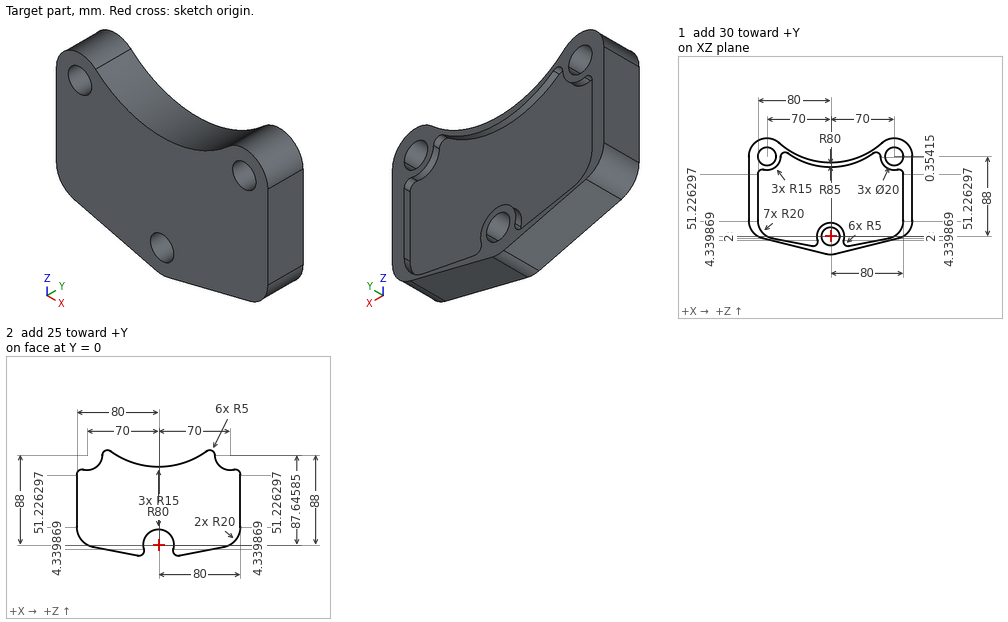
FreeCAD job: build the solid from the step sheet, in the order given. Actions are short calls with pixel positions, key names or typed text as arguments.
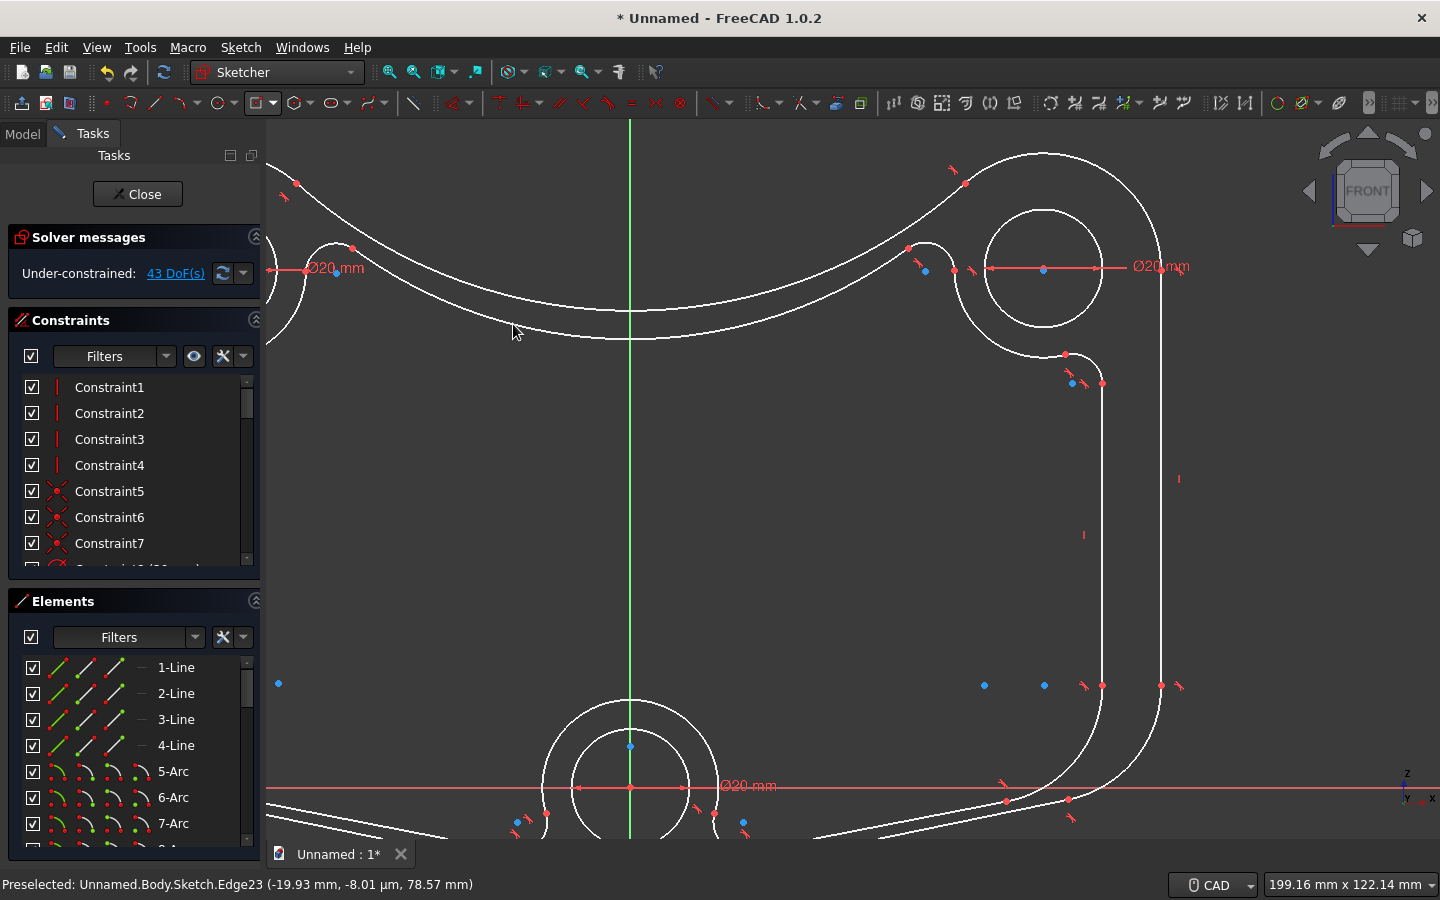
click(513, 324)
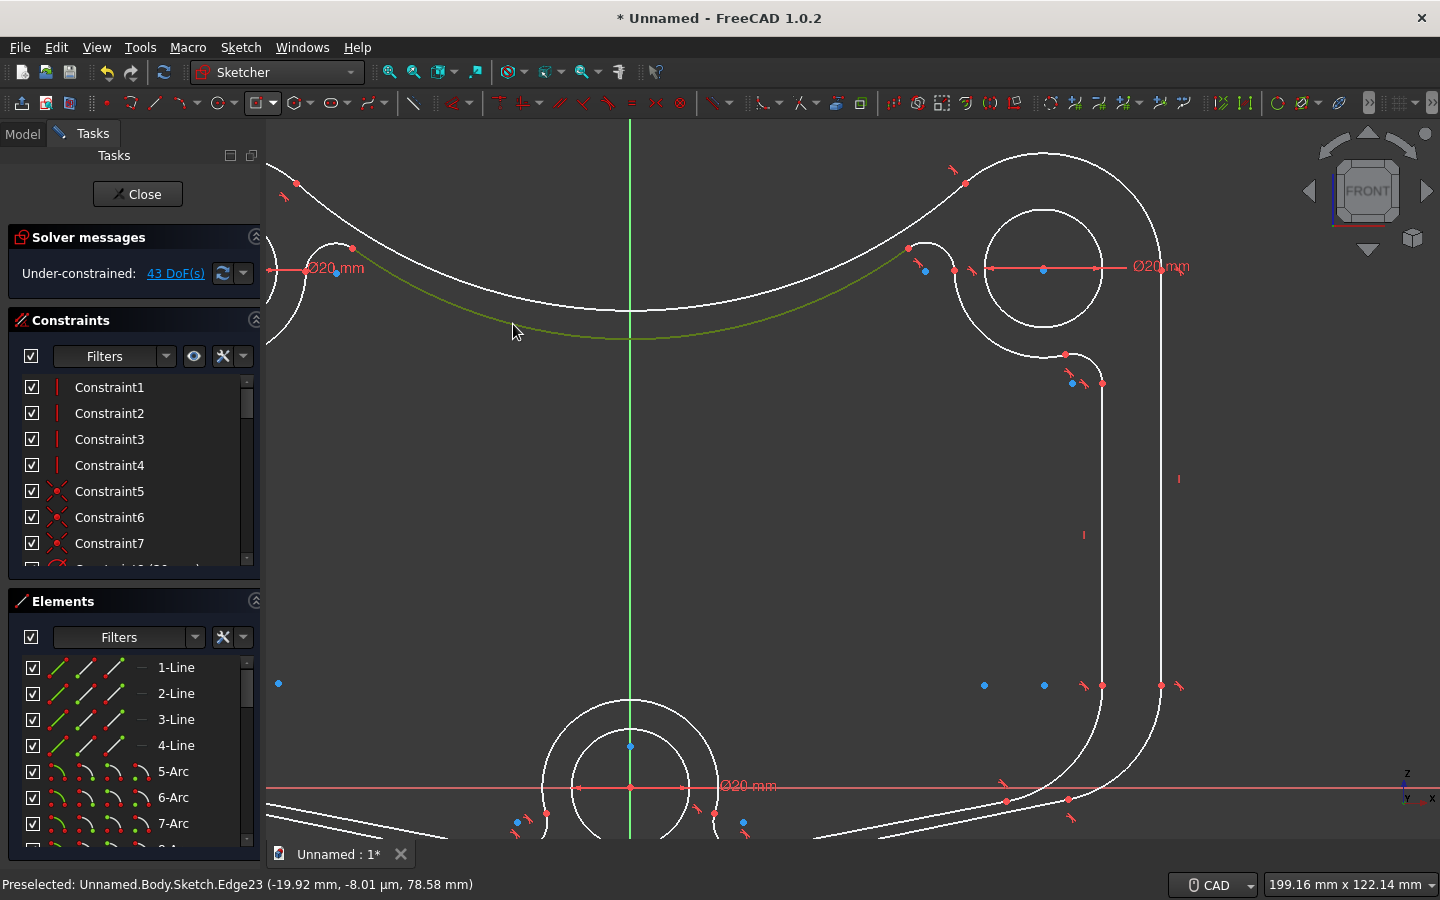
click(335, 243)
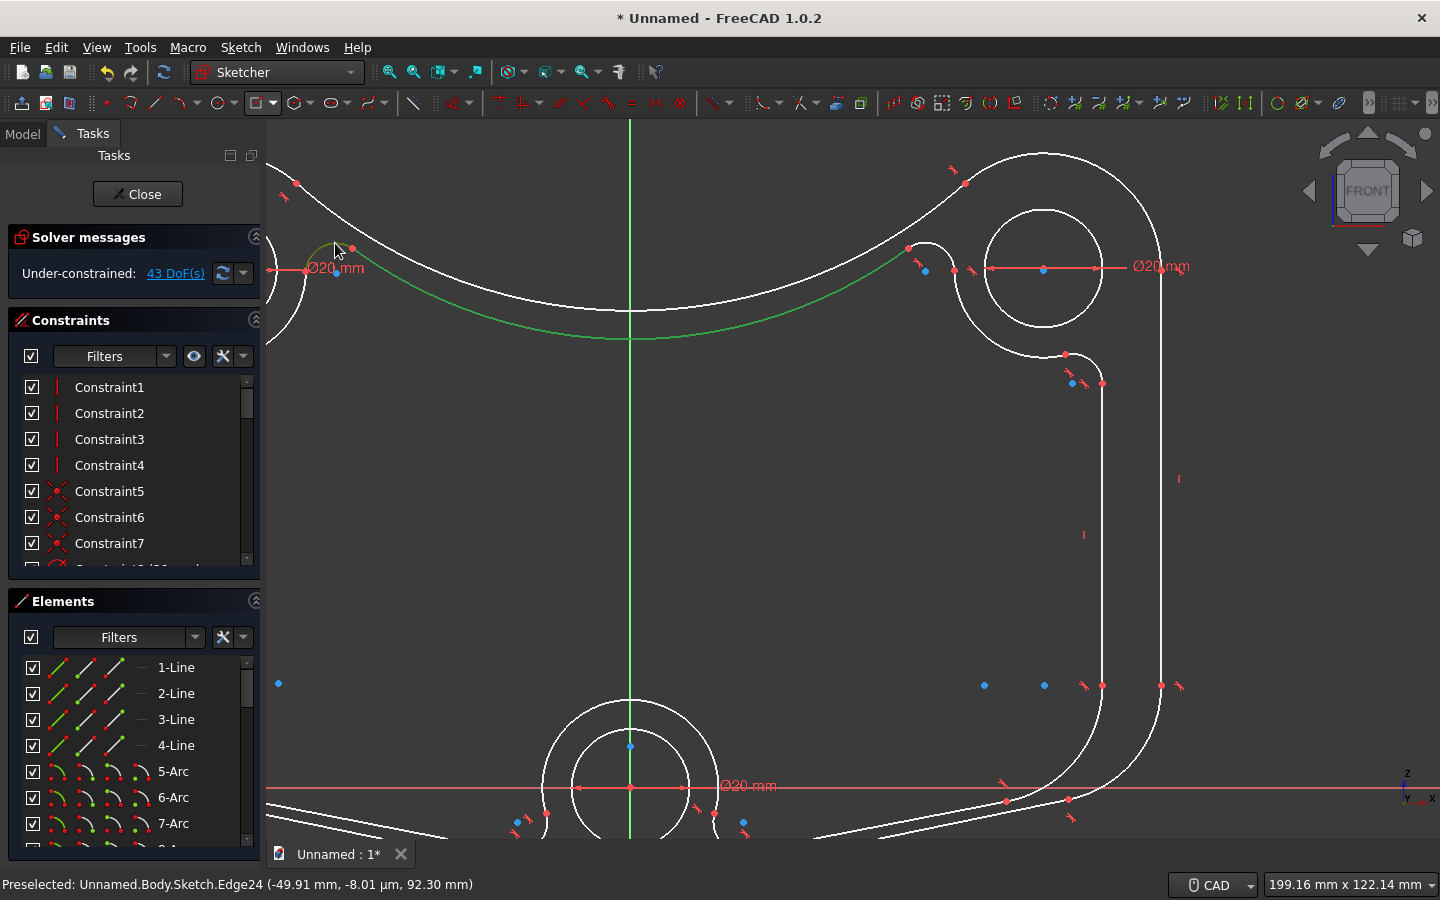
click(608, 104)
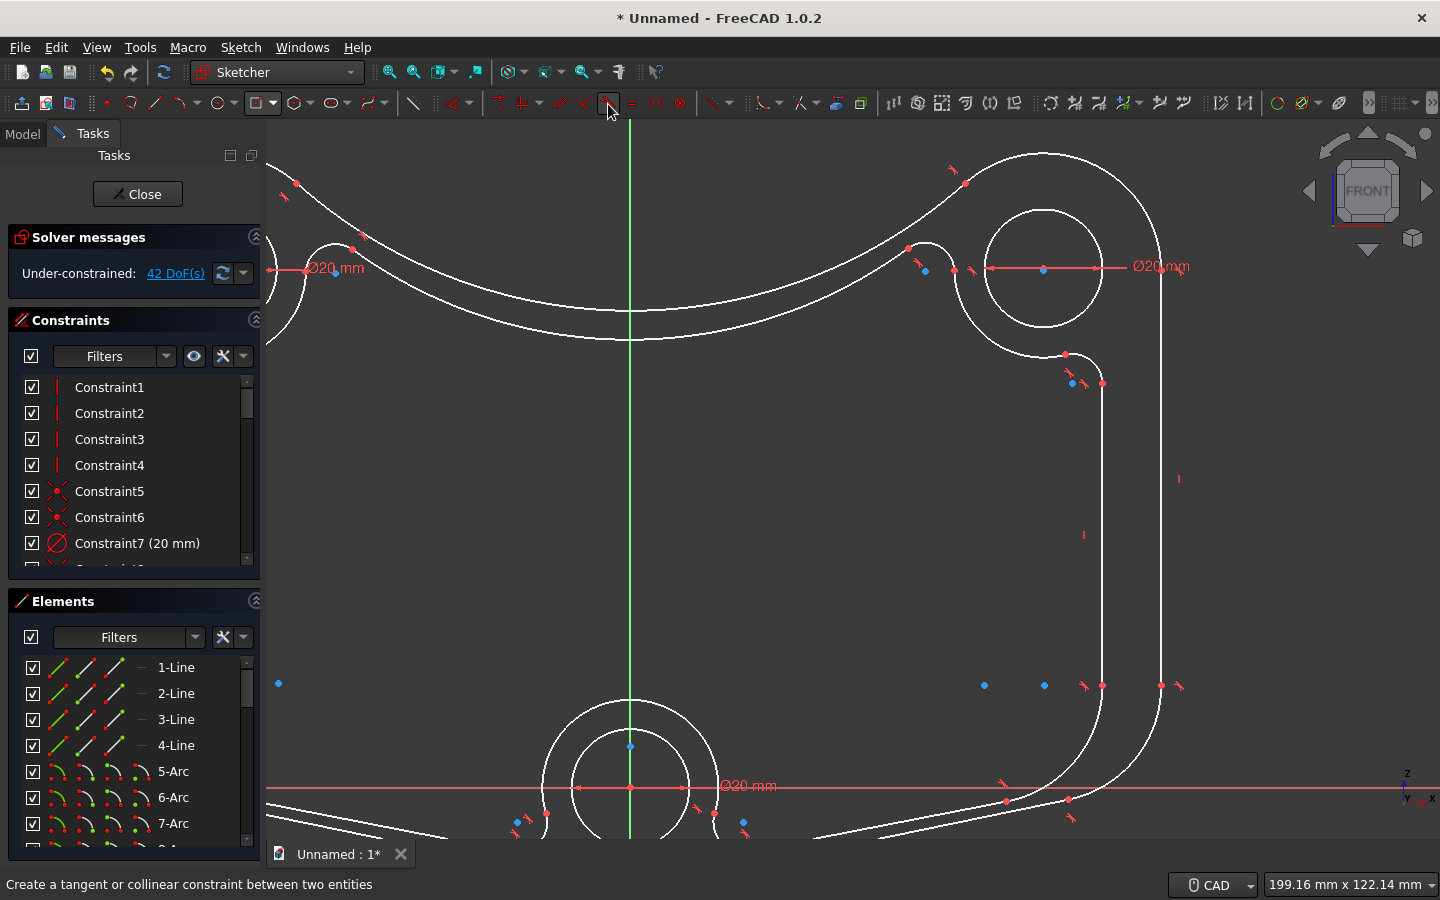
click(335, 244)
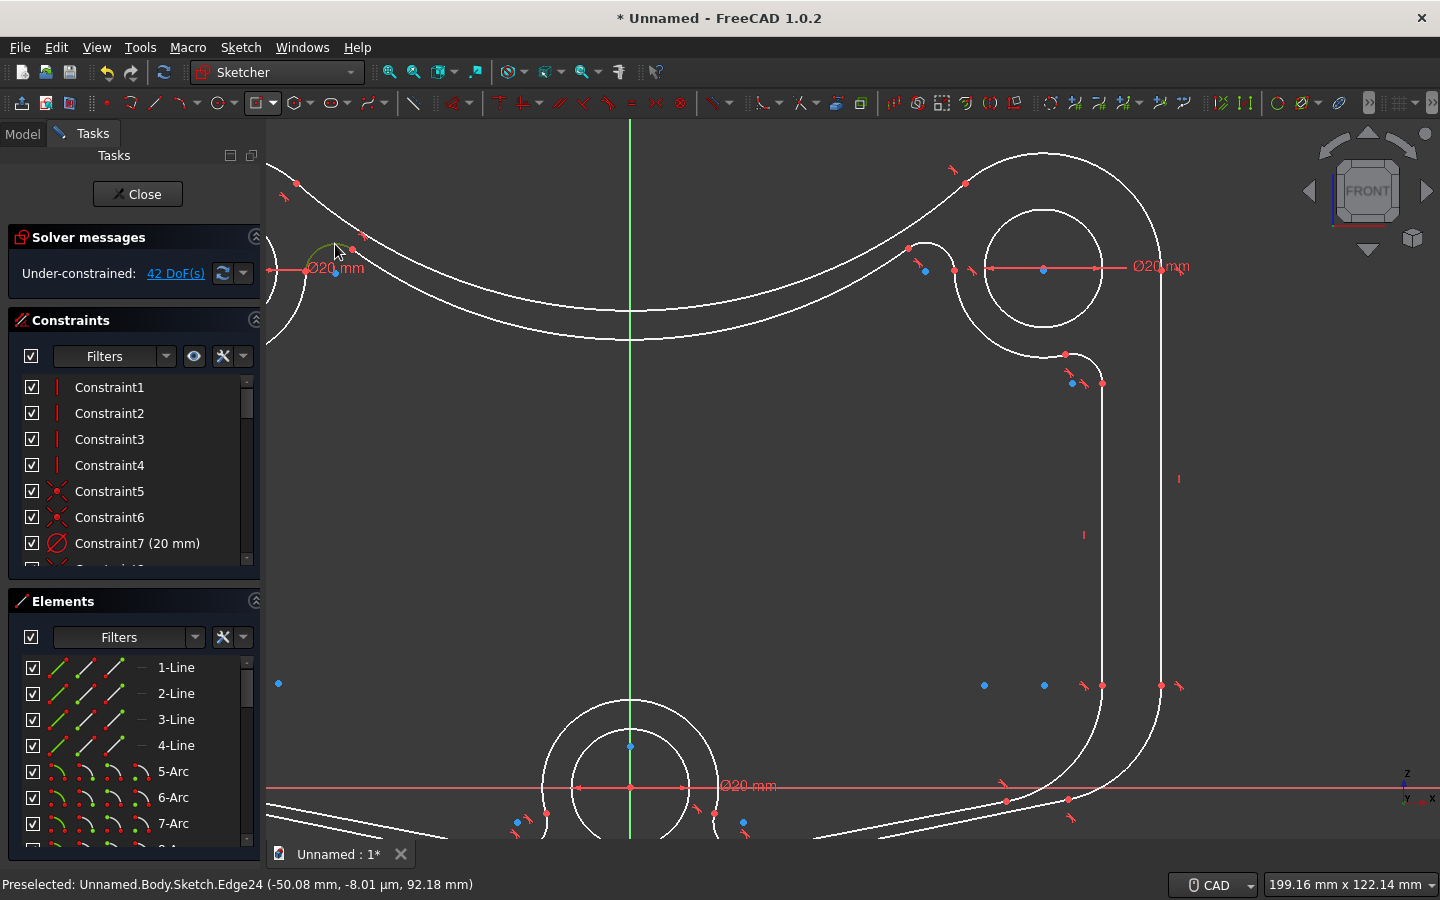
click(300, 303)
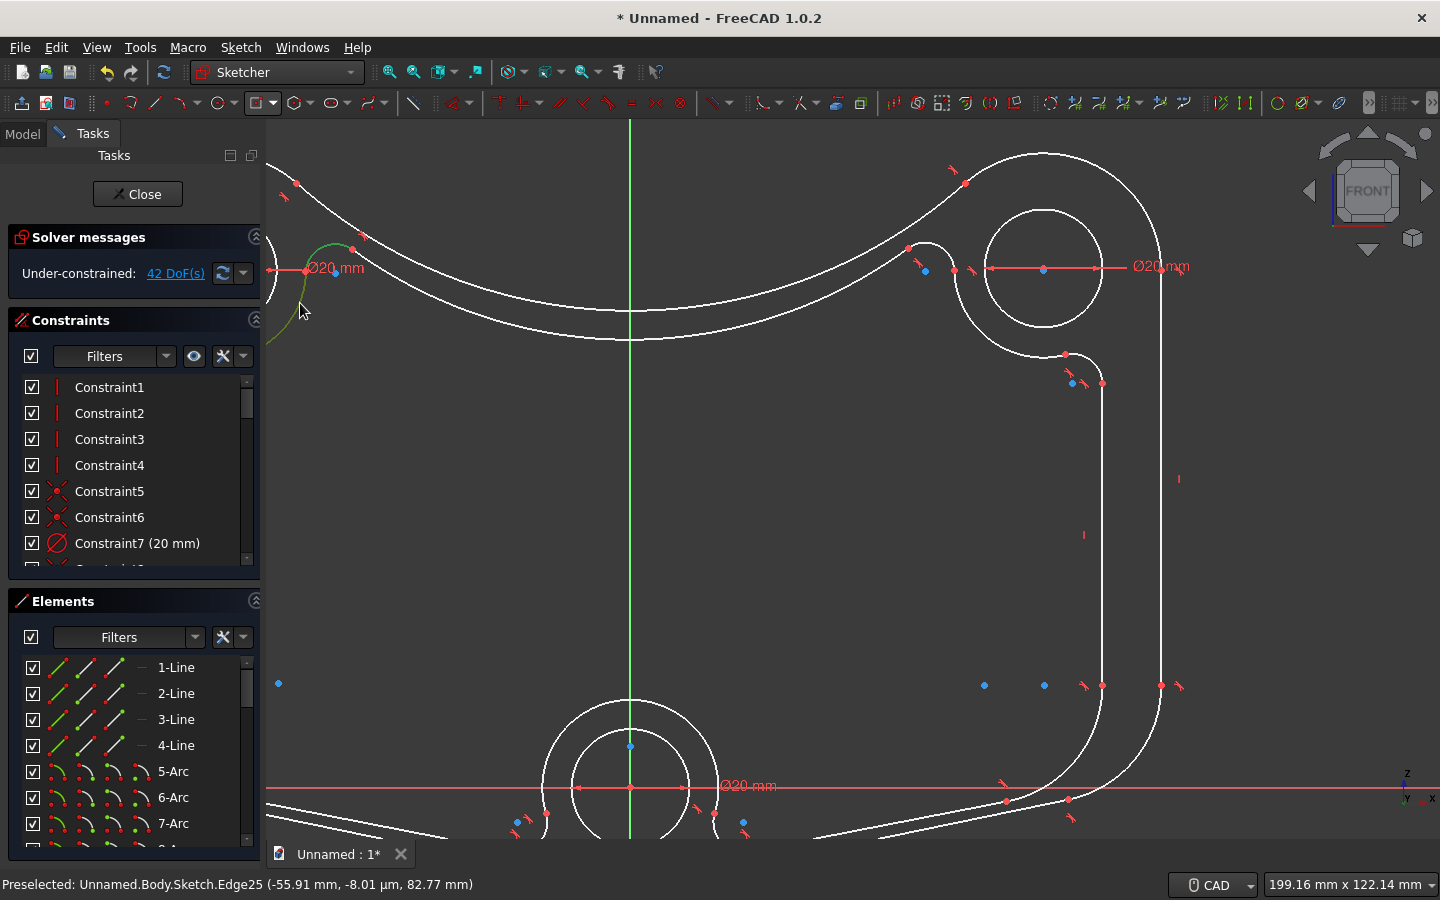
click(608, 104)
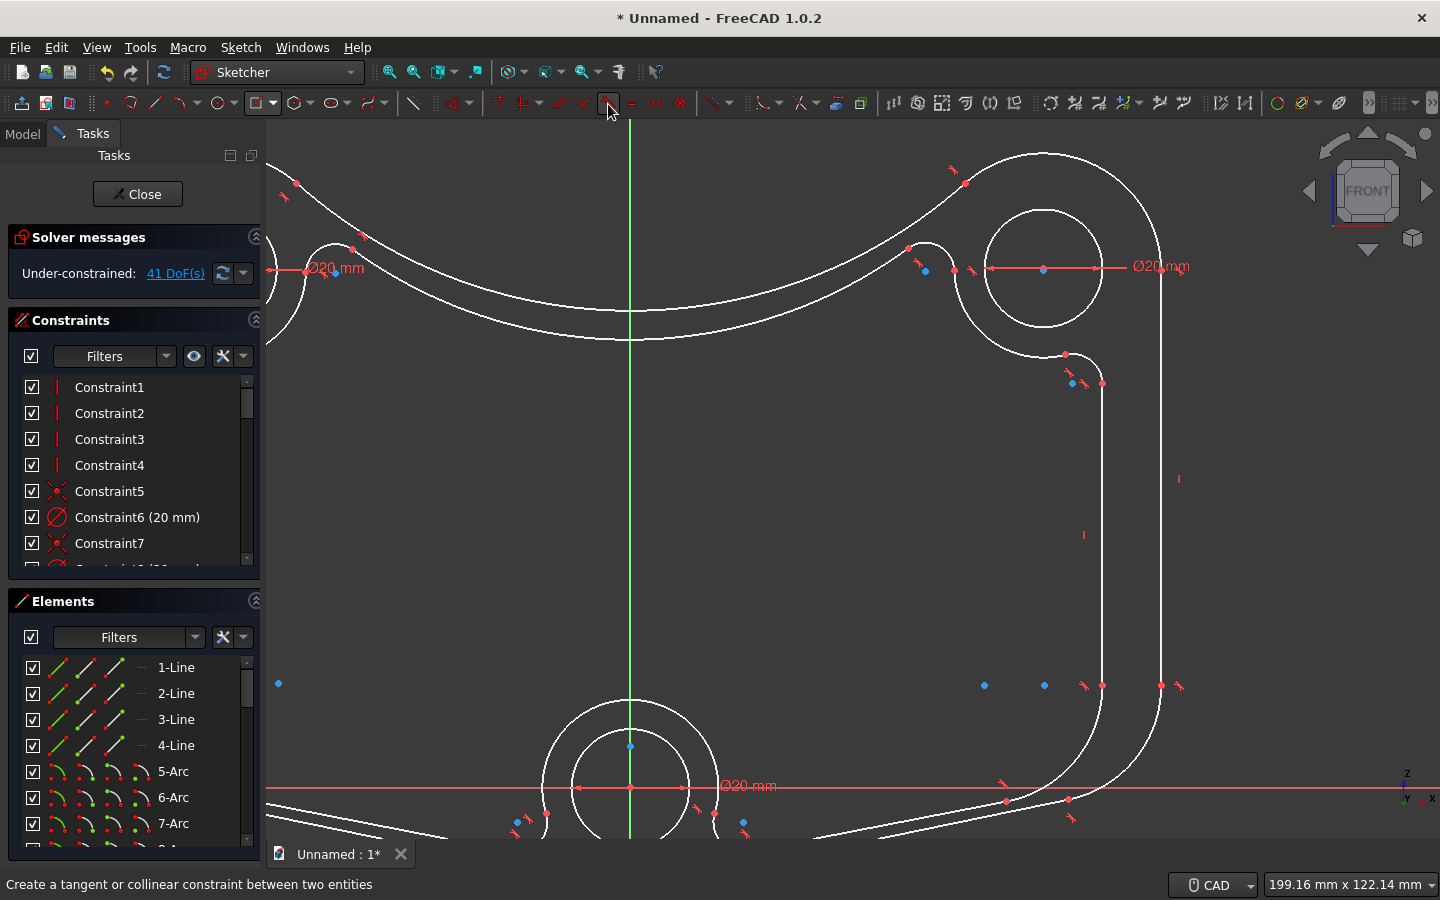
click(299, 304)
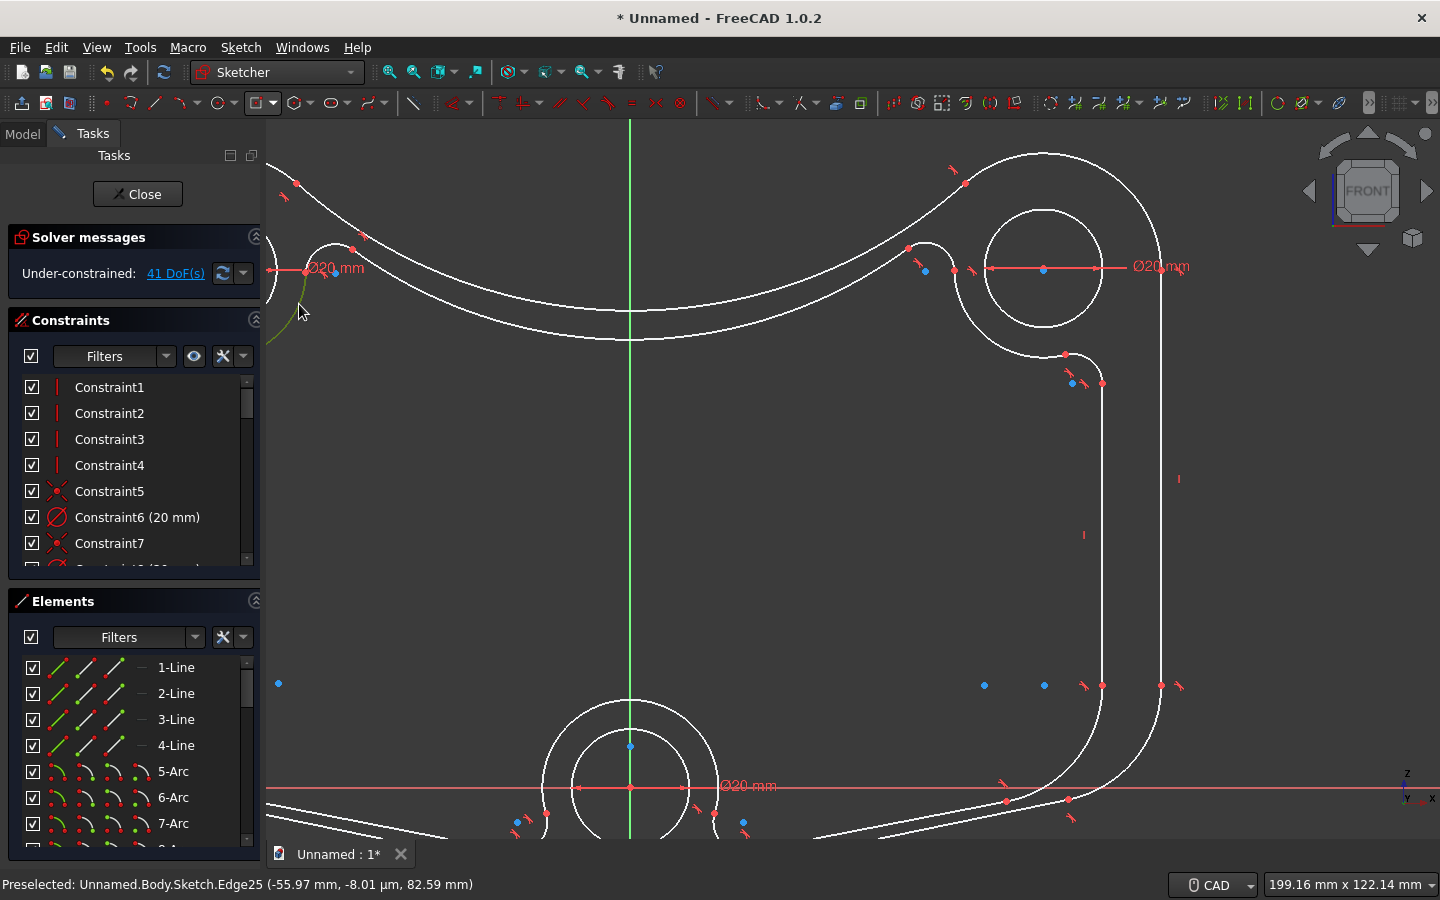
scroll(1098, 369, down, 2)